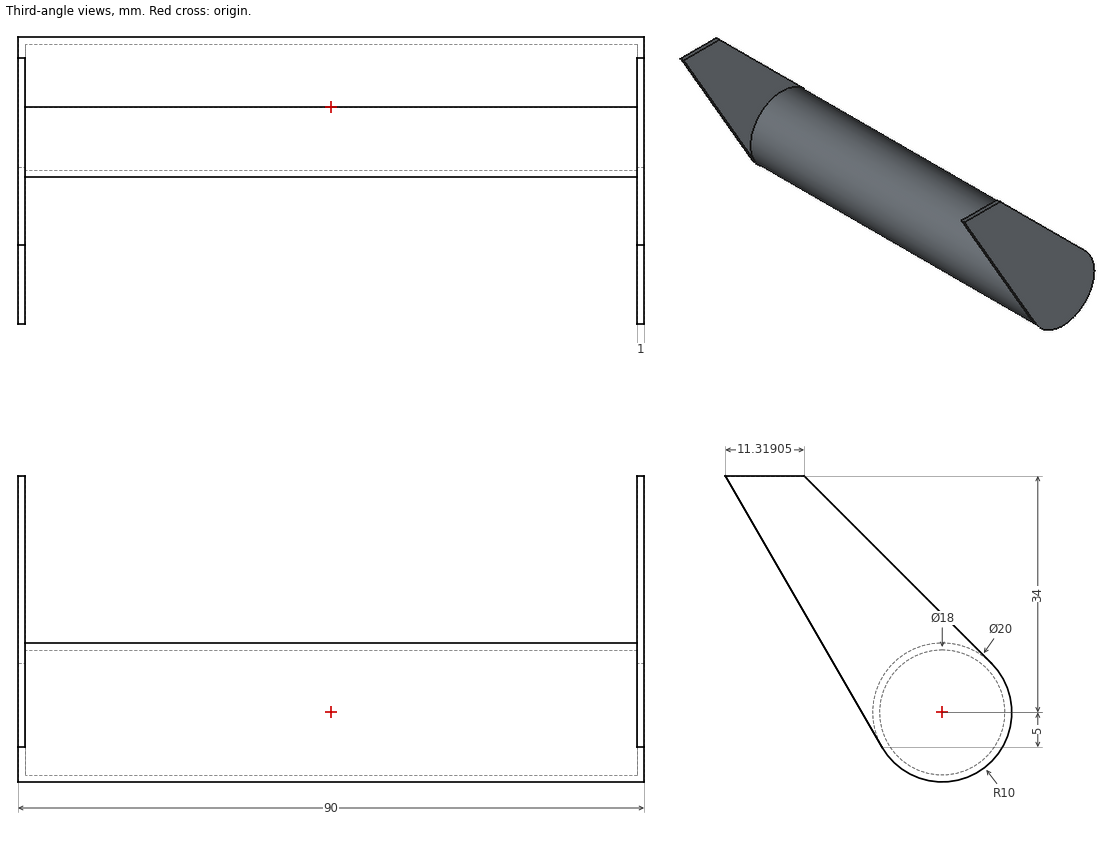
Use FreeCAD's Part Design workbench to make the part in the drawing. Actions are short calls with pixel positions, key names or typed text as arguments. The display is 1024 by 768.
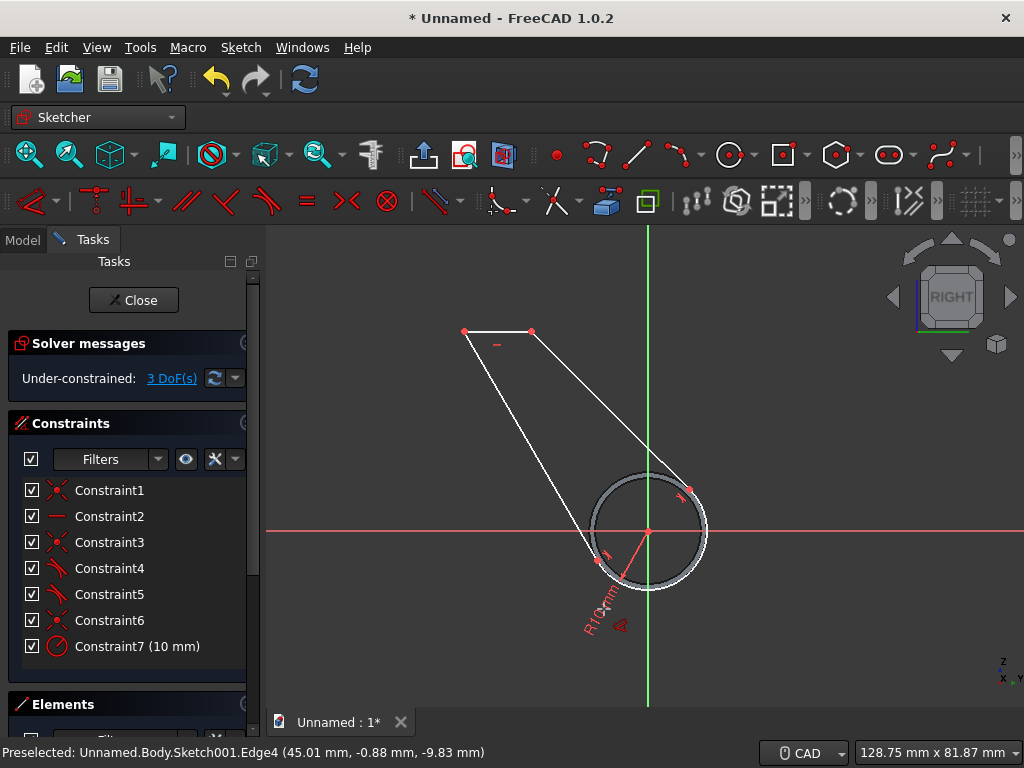
scroll(597, 561, up, 2)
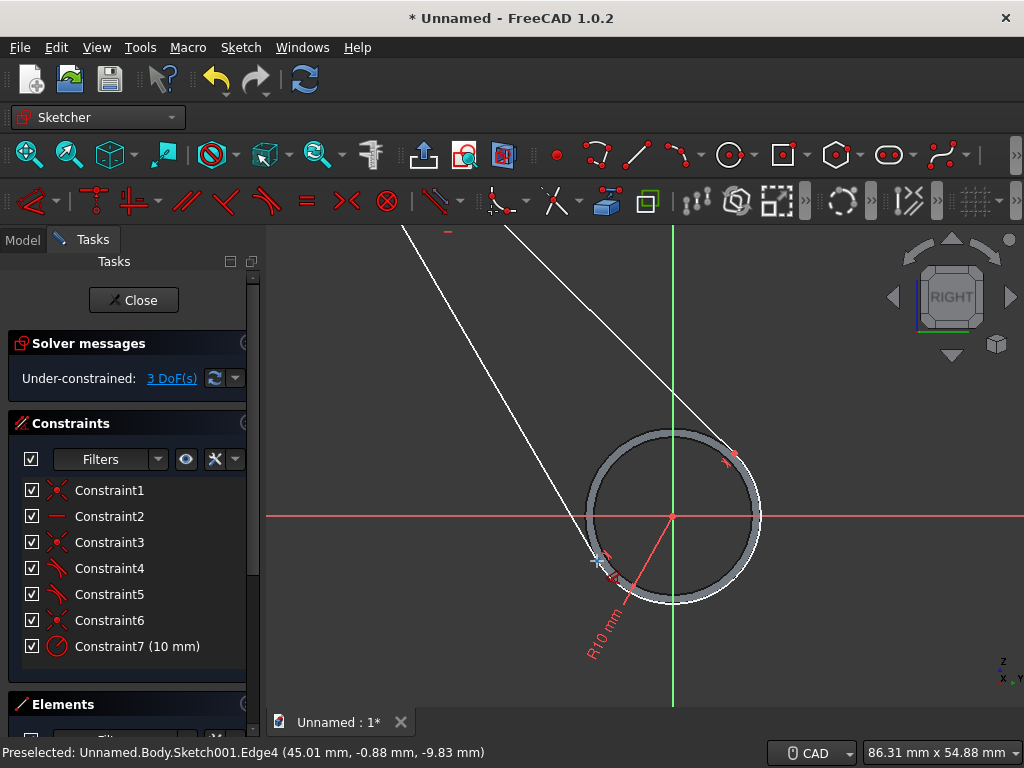
click(597, 560)
click(707, 538)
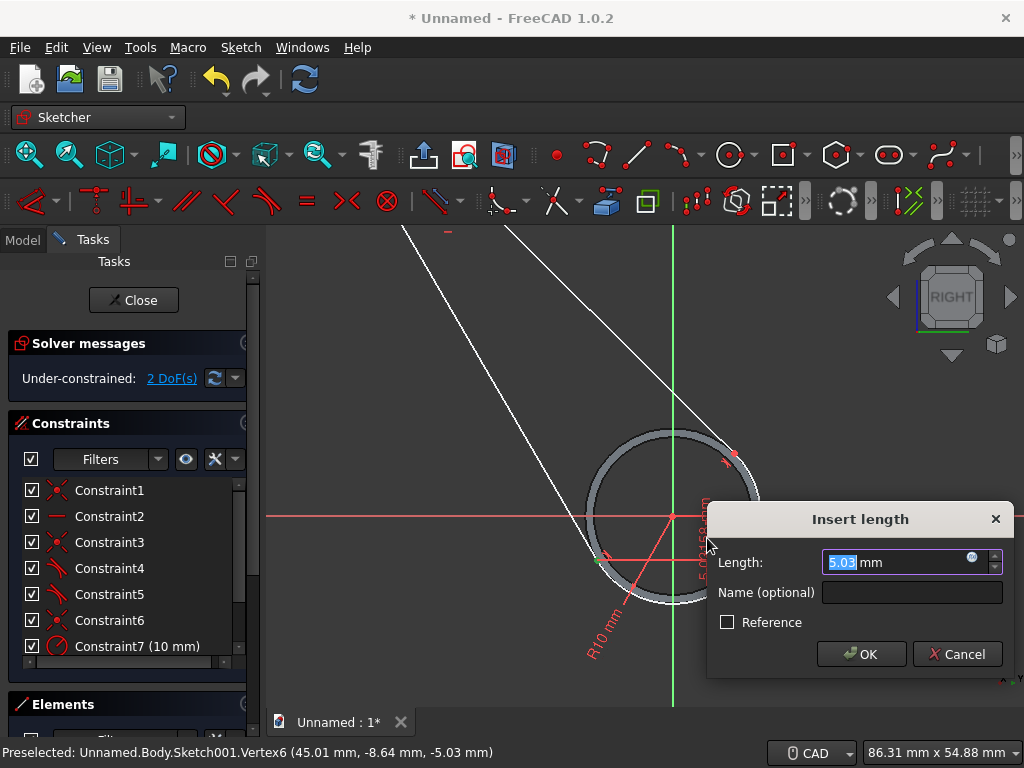
text(5)
key(Return)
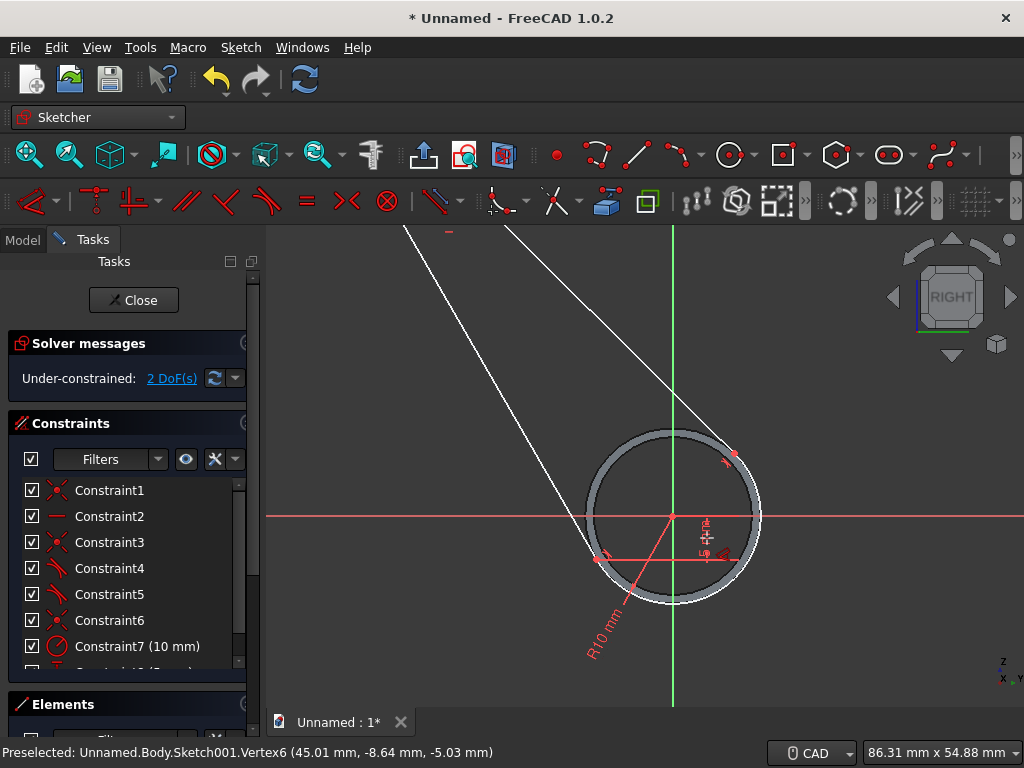
scroll(619, 679, down, 1)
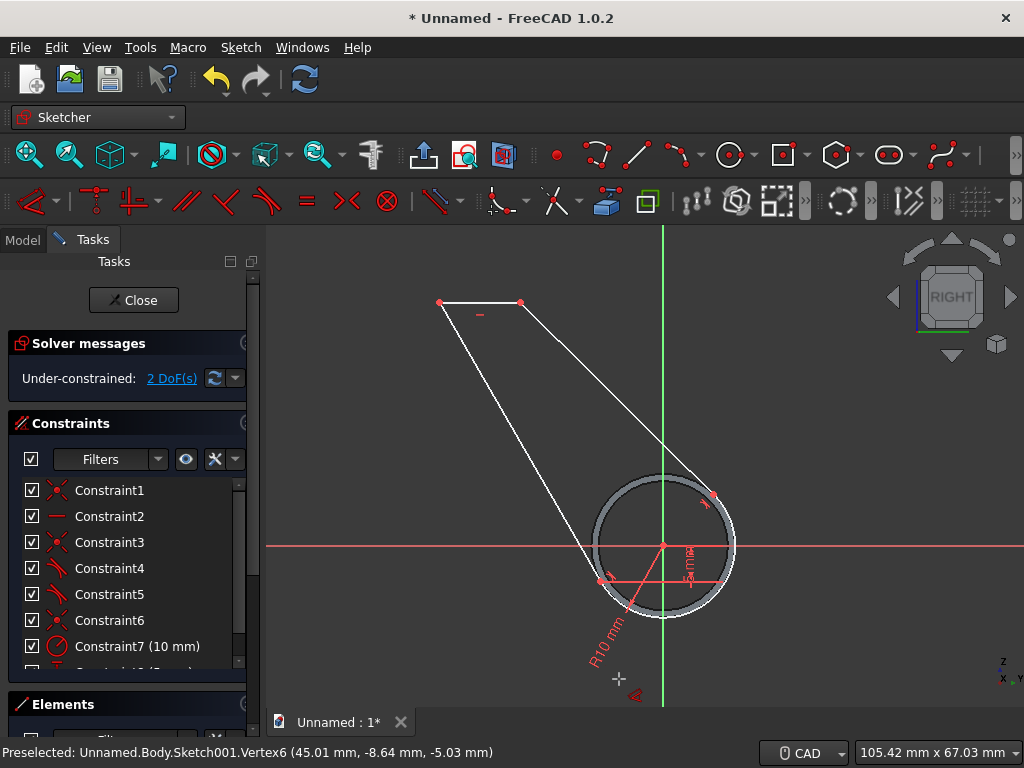
click(520, 303)
click(697, 424)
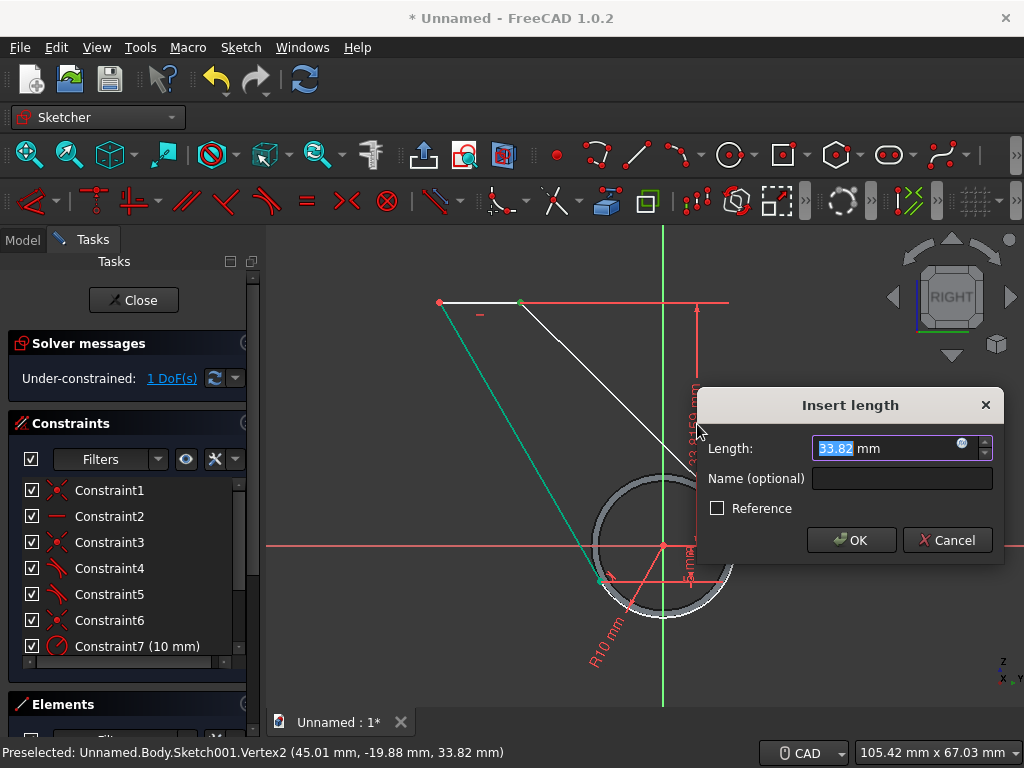
text(34)
key(Return)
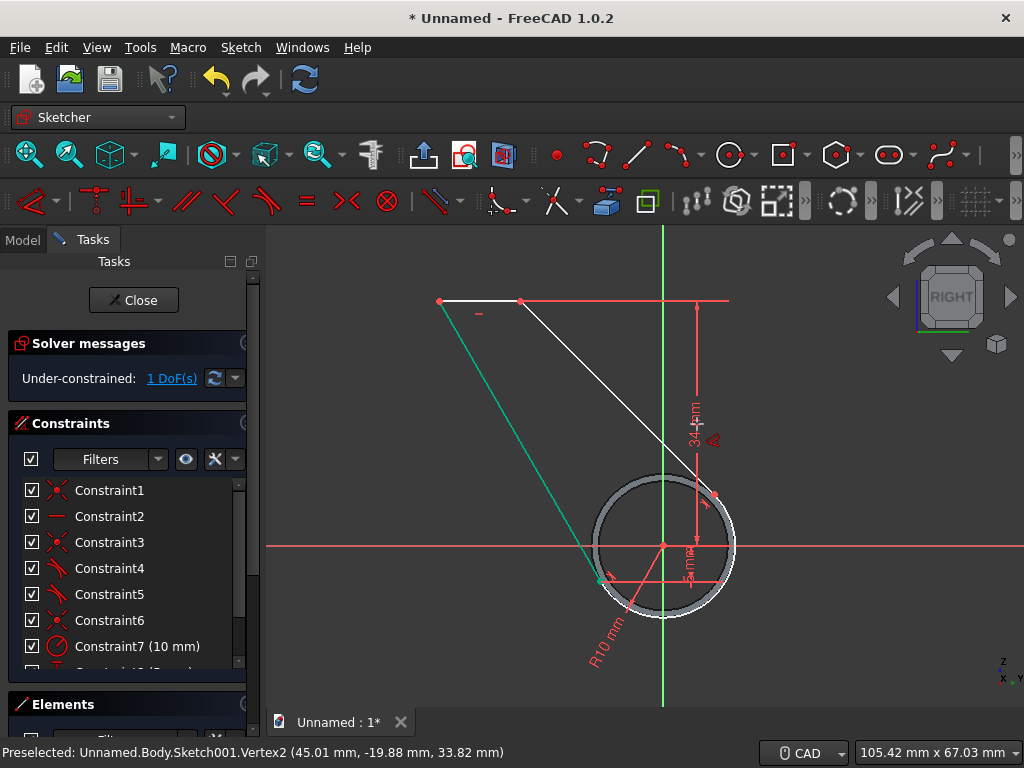
click(496, 301)
click(480, 267)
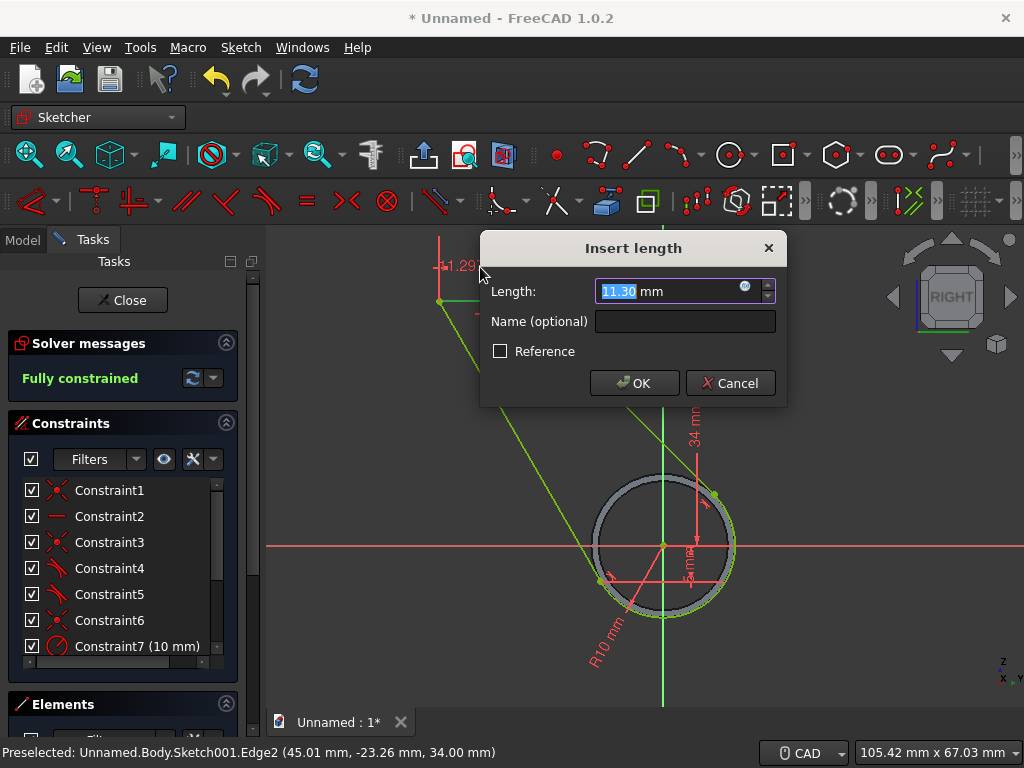
text(11.31905)
key(Return)
key(Escape)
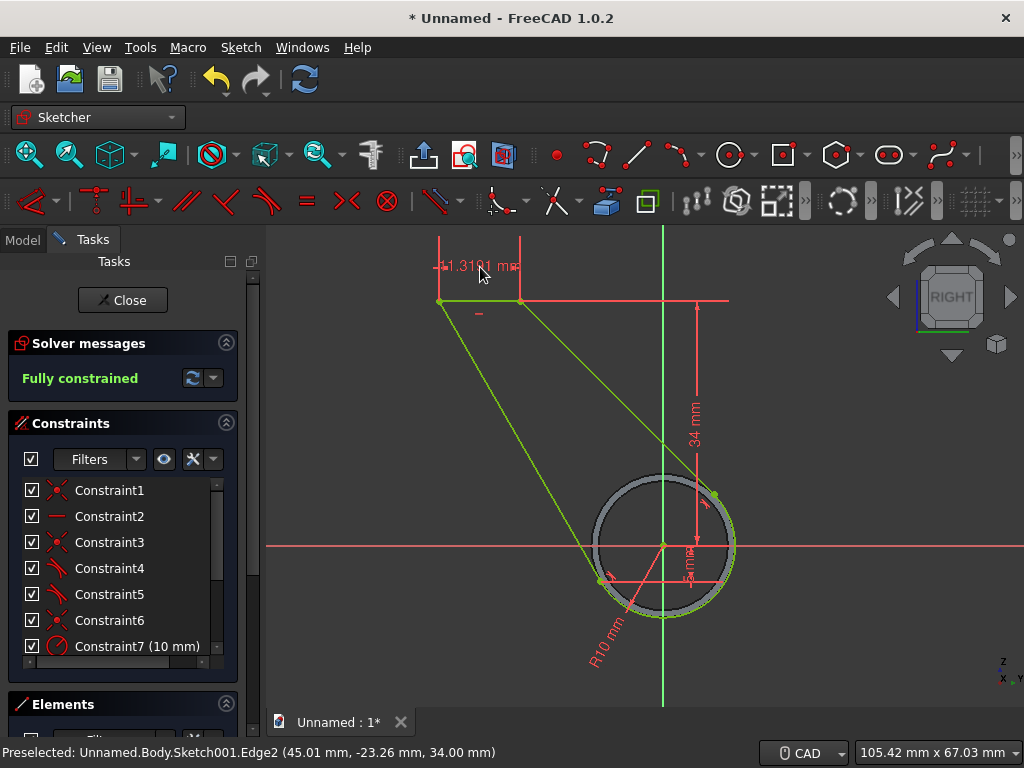
click(123, 300)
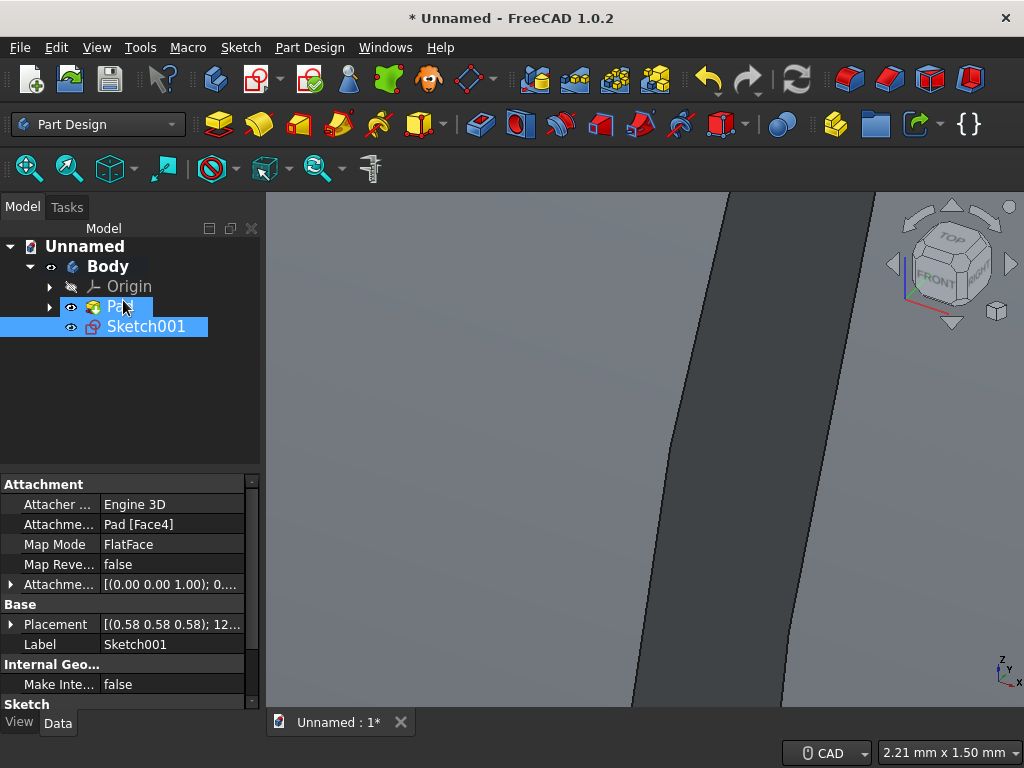
click(220, 124)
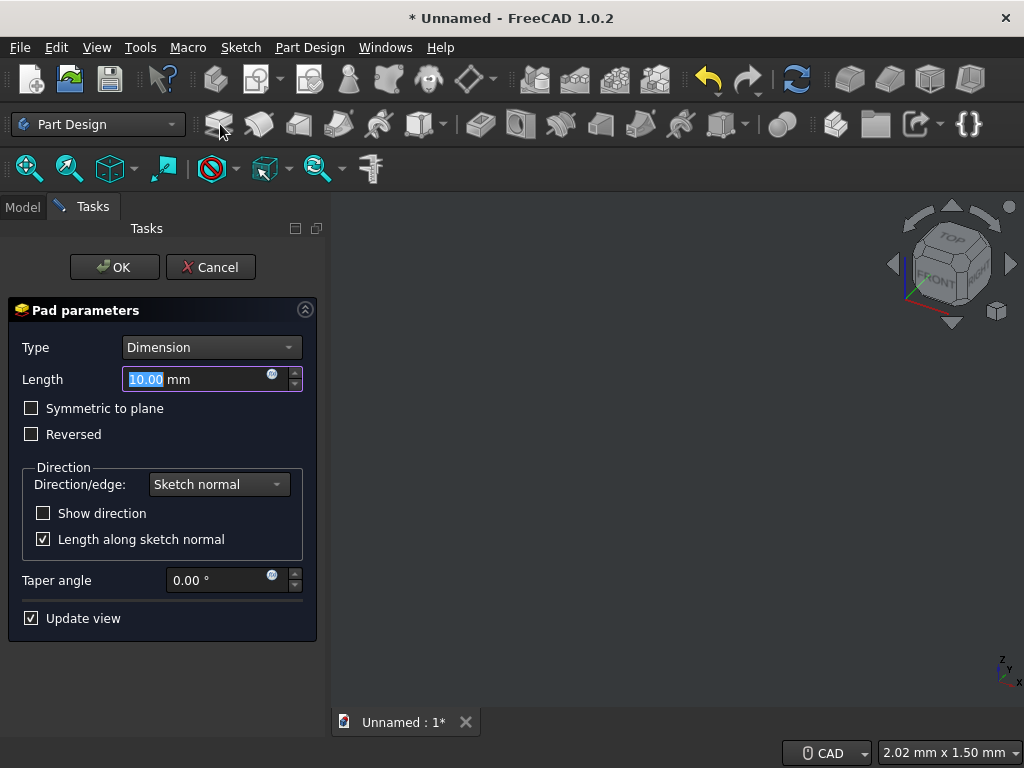
text(1)
key(Tab)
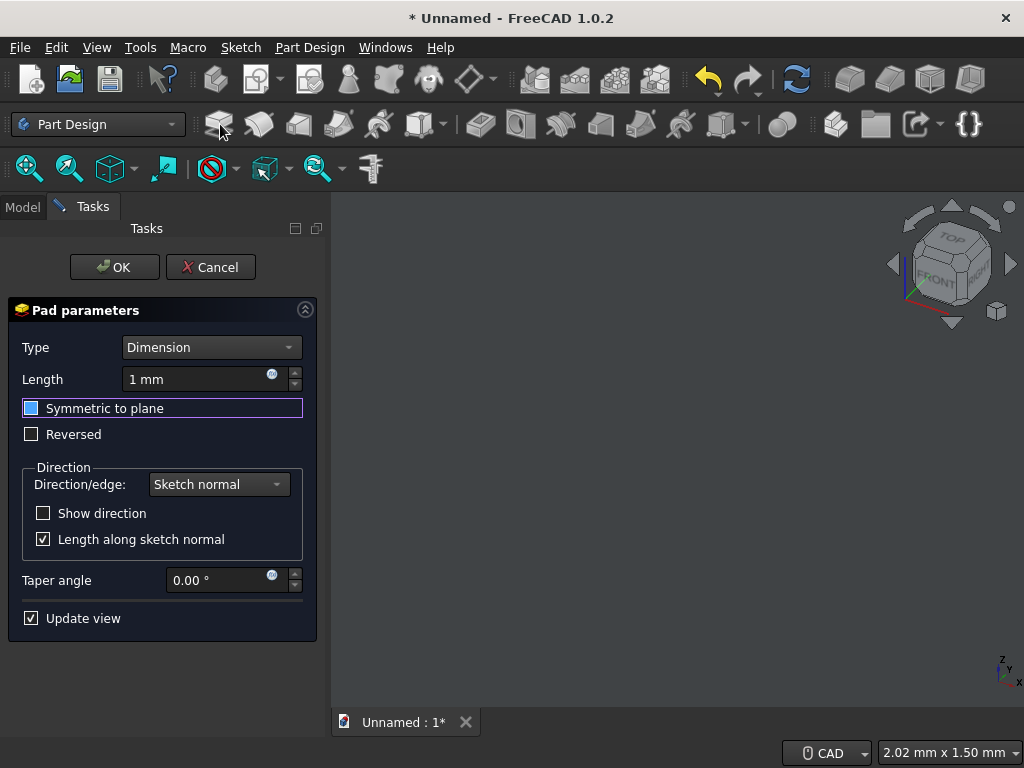
click(30, 434)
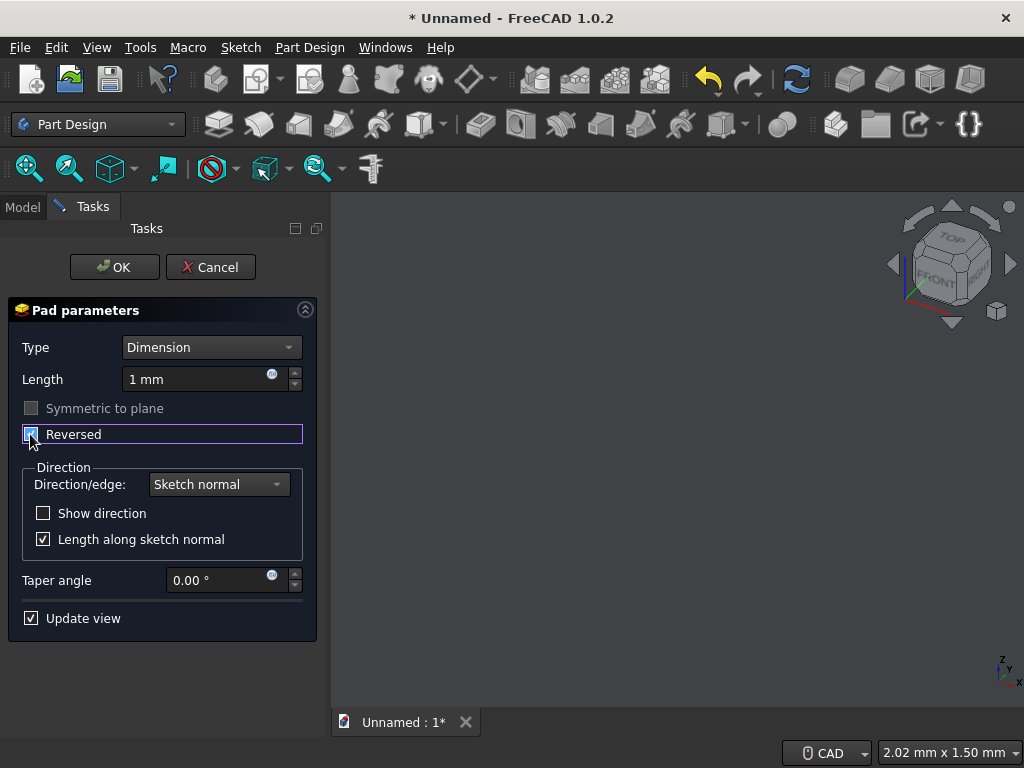
click(115, 267)